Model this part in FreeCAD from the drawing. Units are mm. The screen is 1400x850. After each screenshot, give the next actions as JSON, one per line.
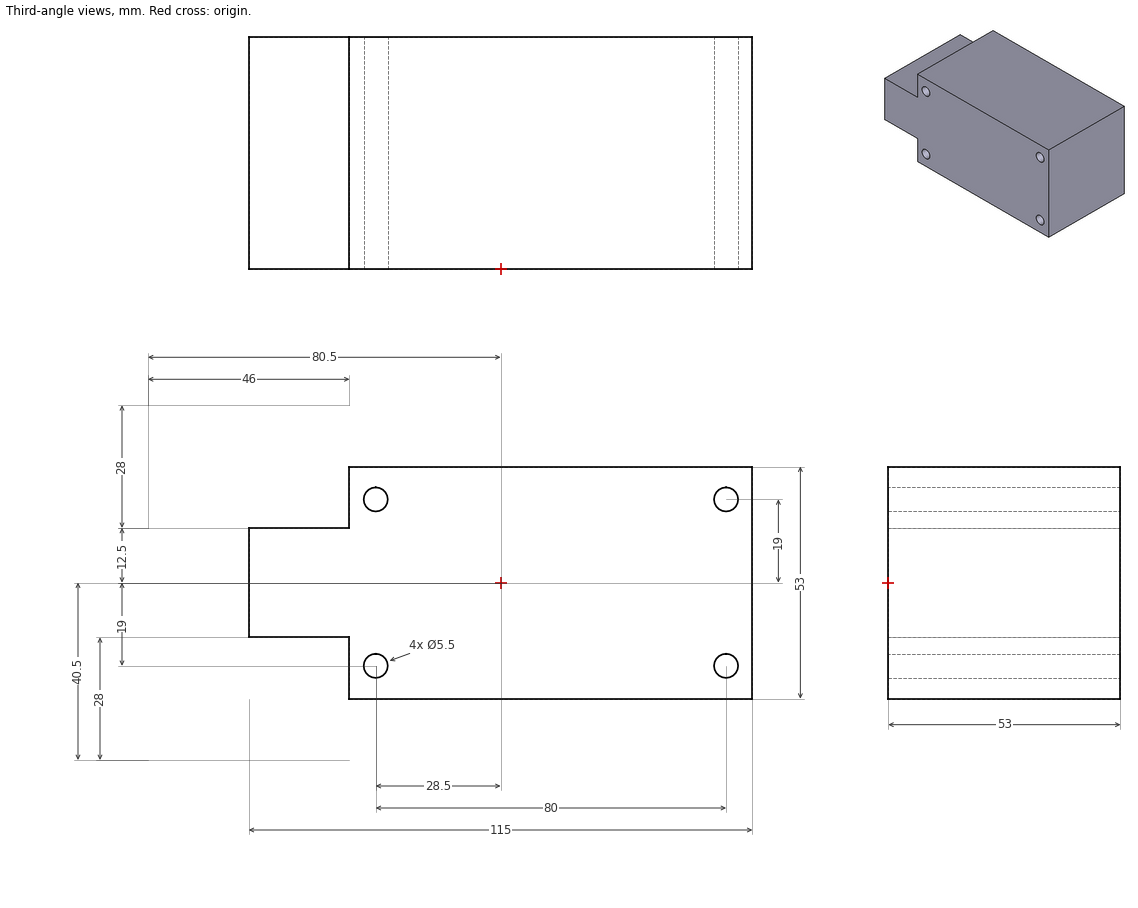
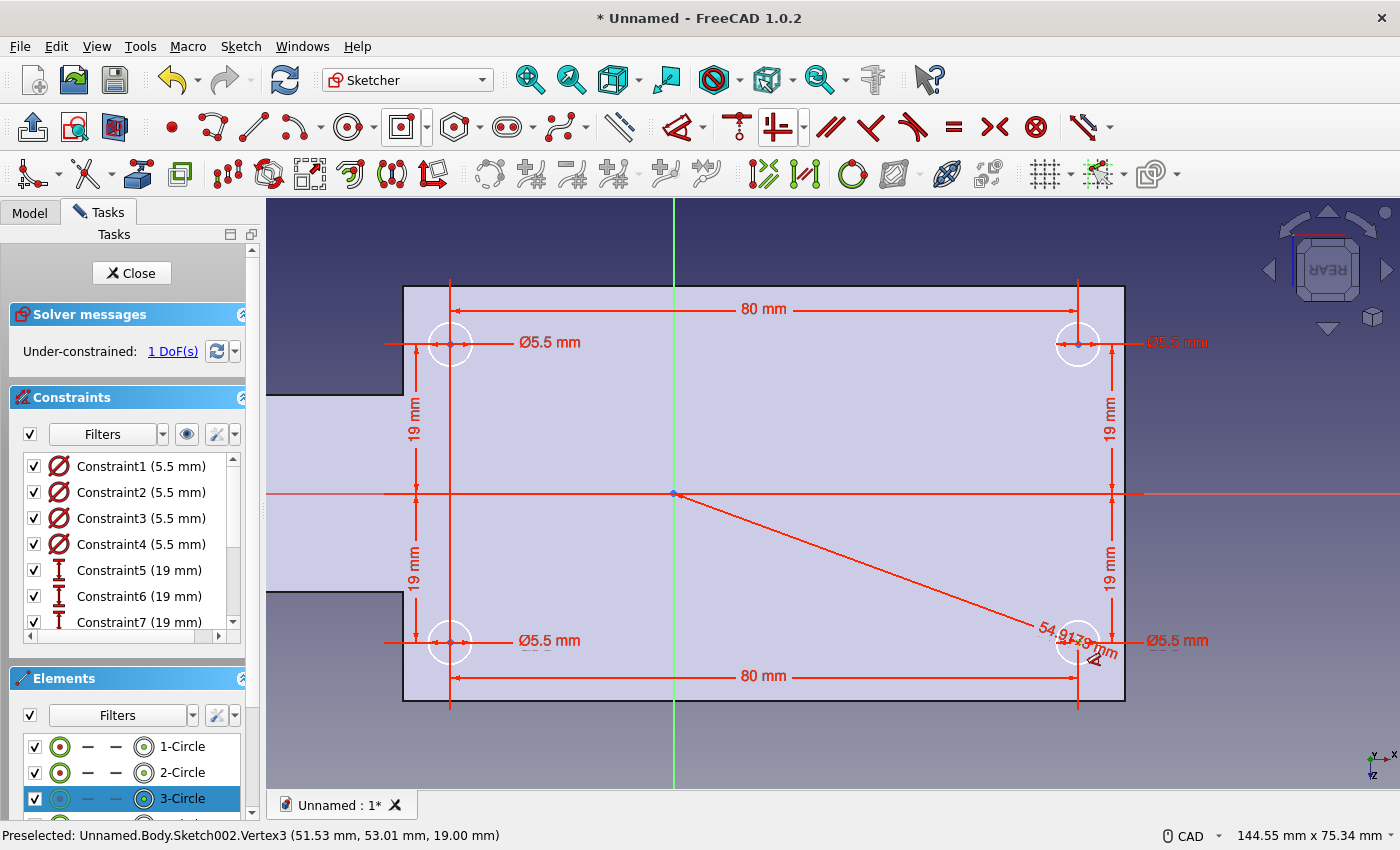
{"action": "left_click", "coordinate": [450, 643]}
{"action": "left_click", "coordinate": [620, 677]}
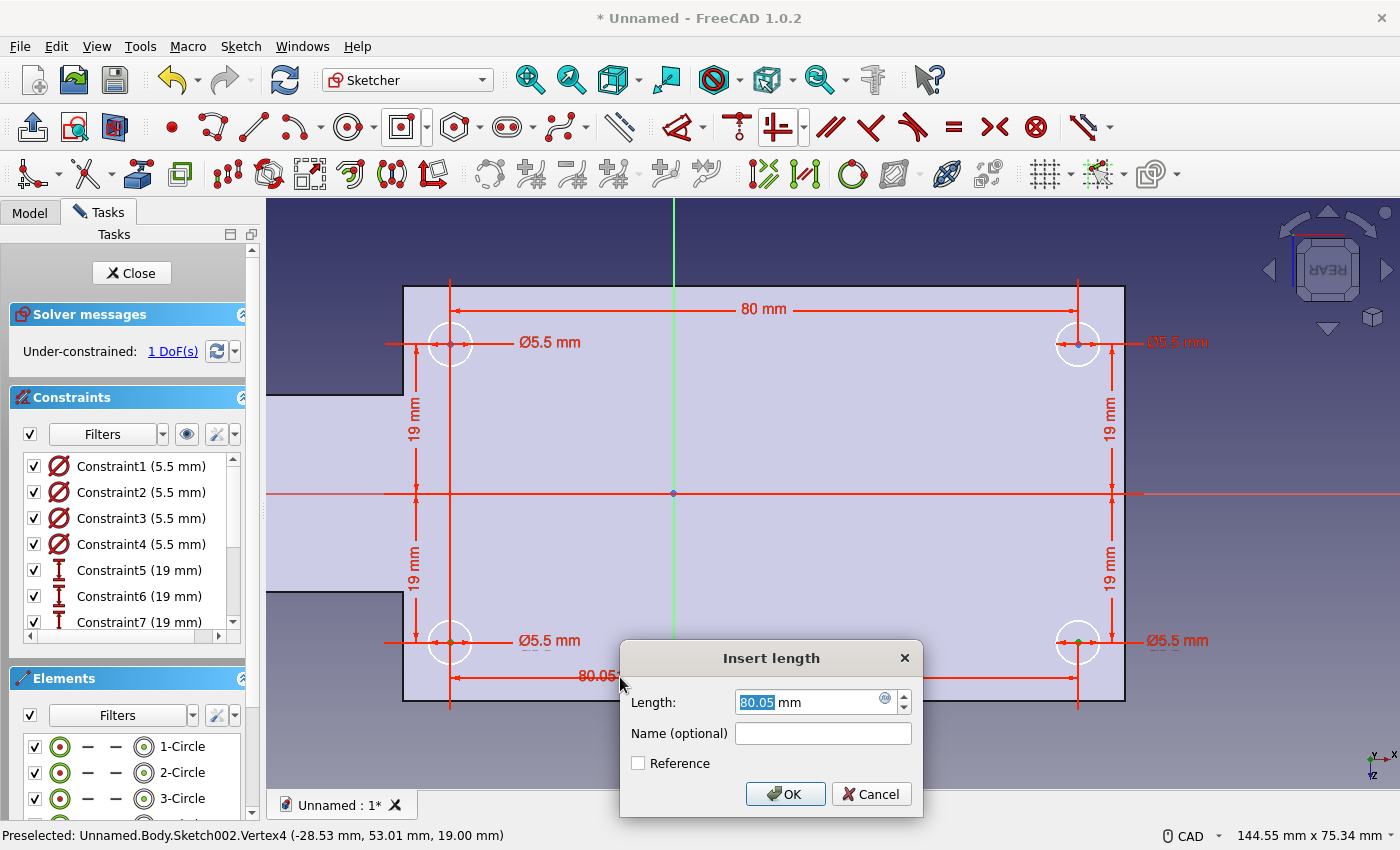
{"action": "type", "text": "80"}
{"action": "key", "text": "Return"}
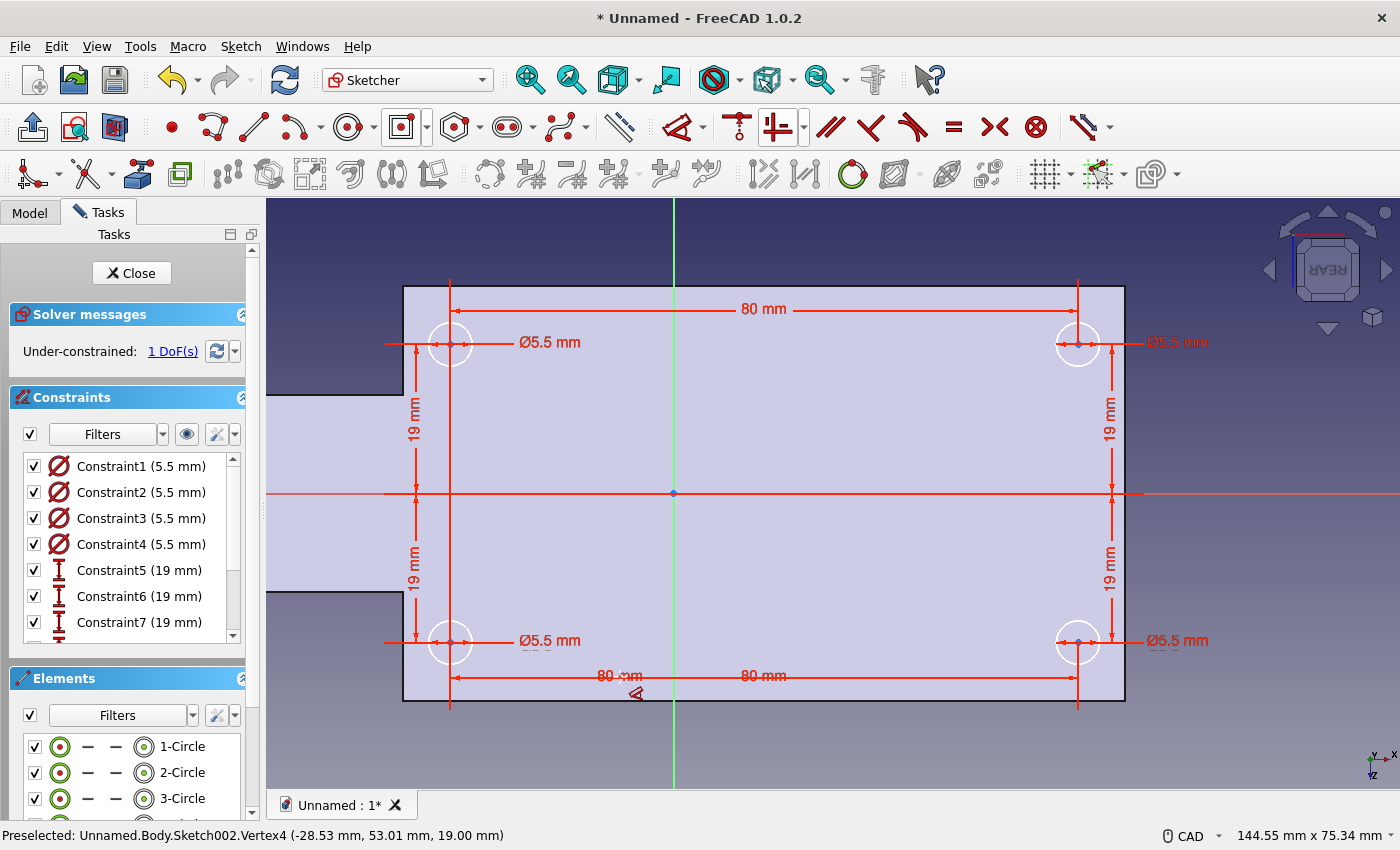
{"action": "left_click", "coordinate": [450, 344]}
{"action": "left_click", "coordinate": [562, 310]}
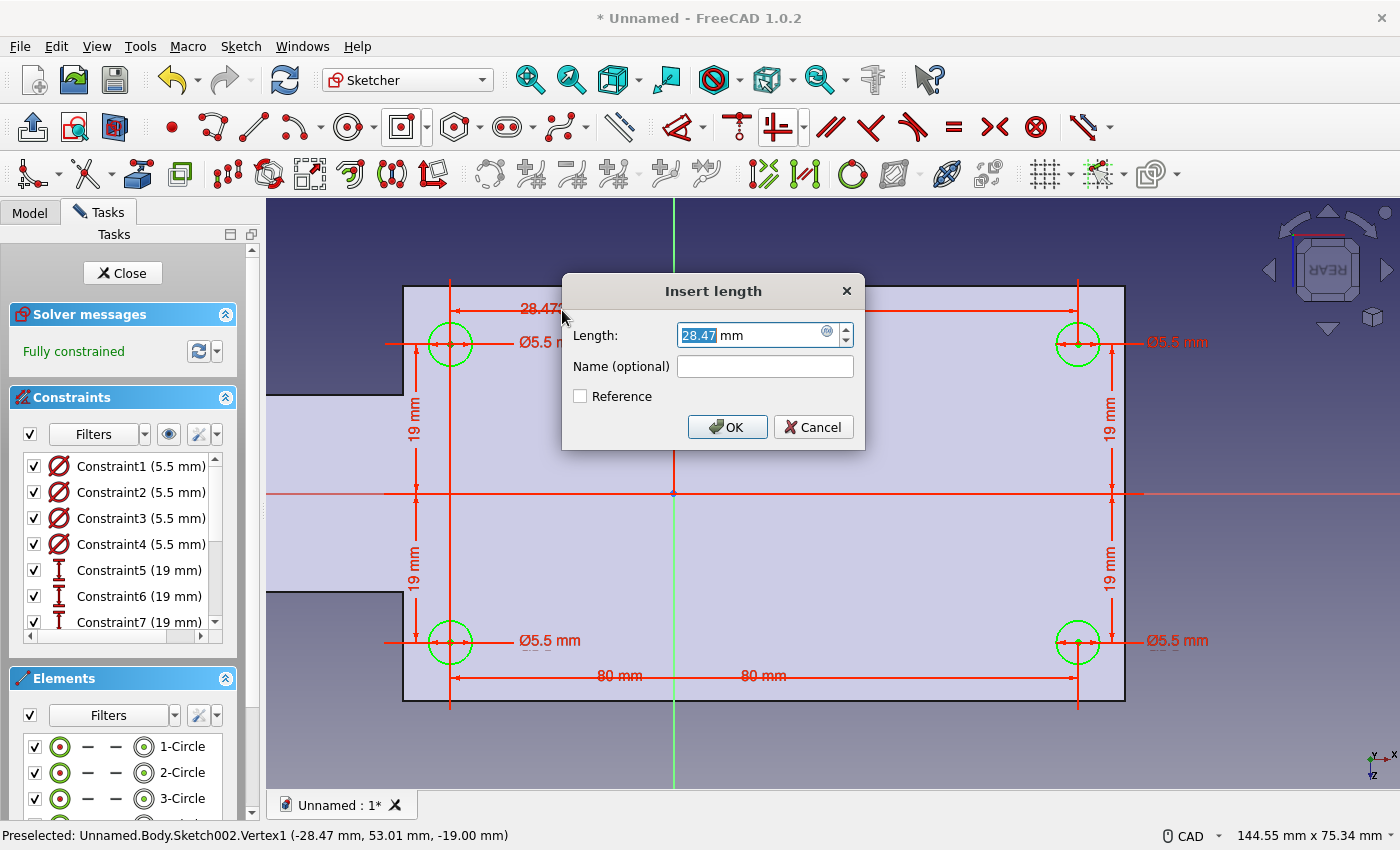
{"action": "type", "text": "28.5"}
{"action": "key", "text": "Return"}
{"action": "key", "text": "Escape"}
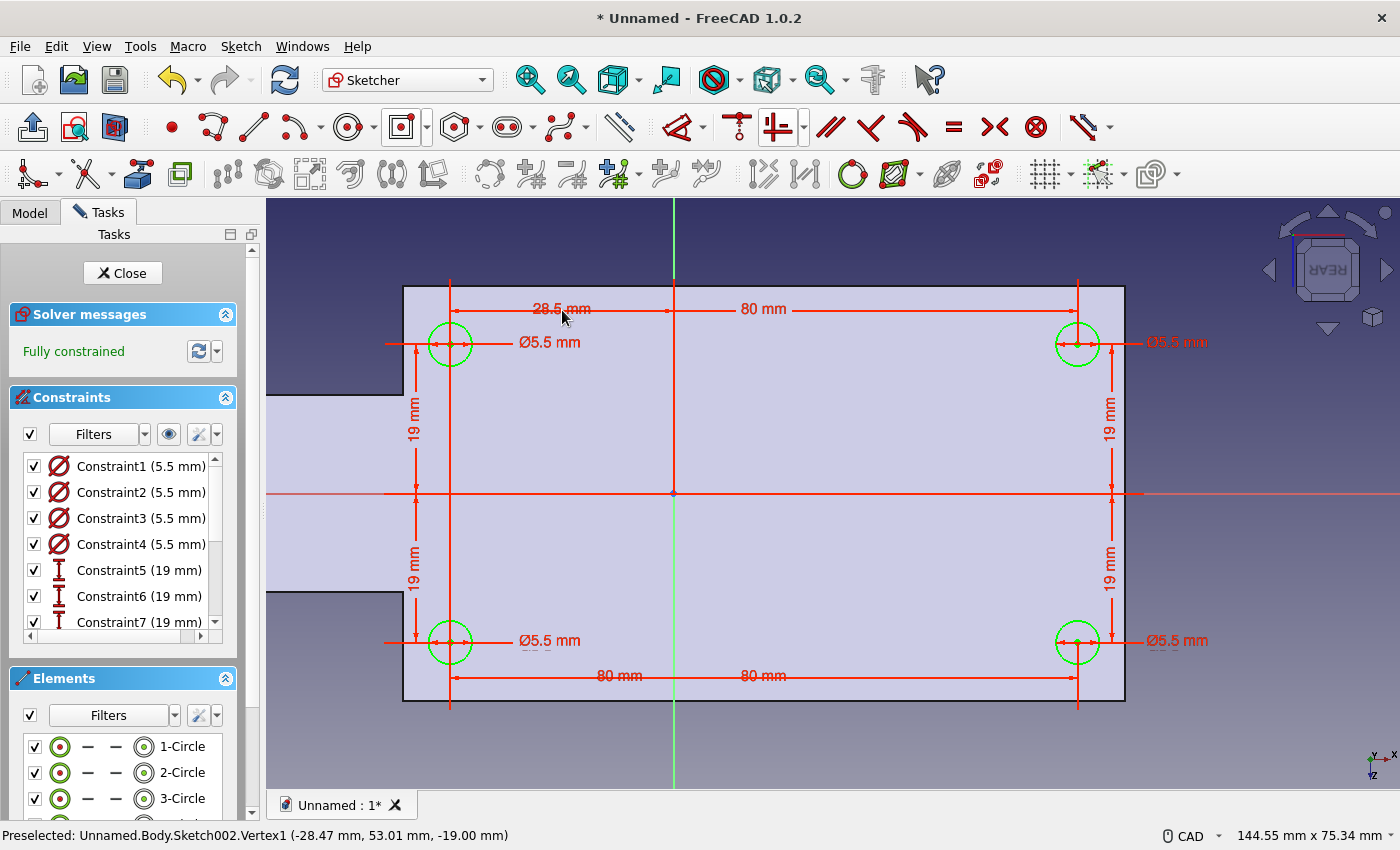
{"action": "left_click", "coordinate": [123, 273]}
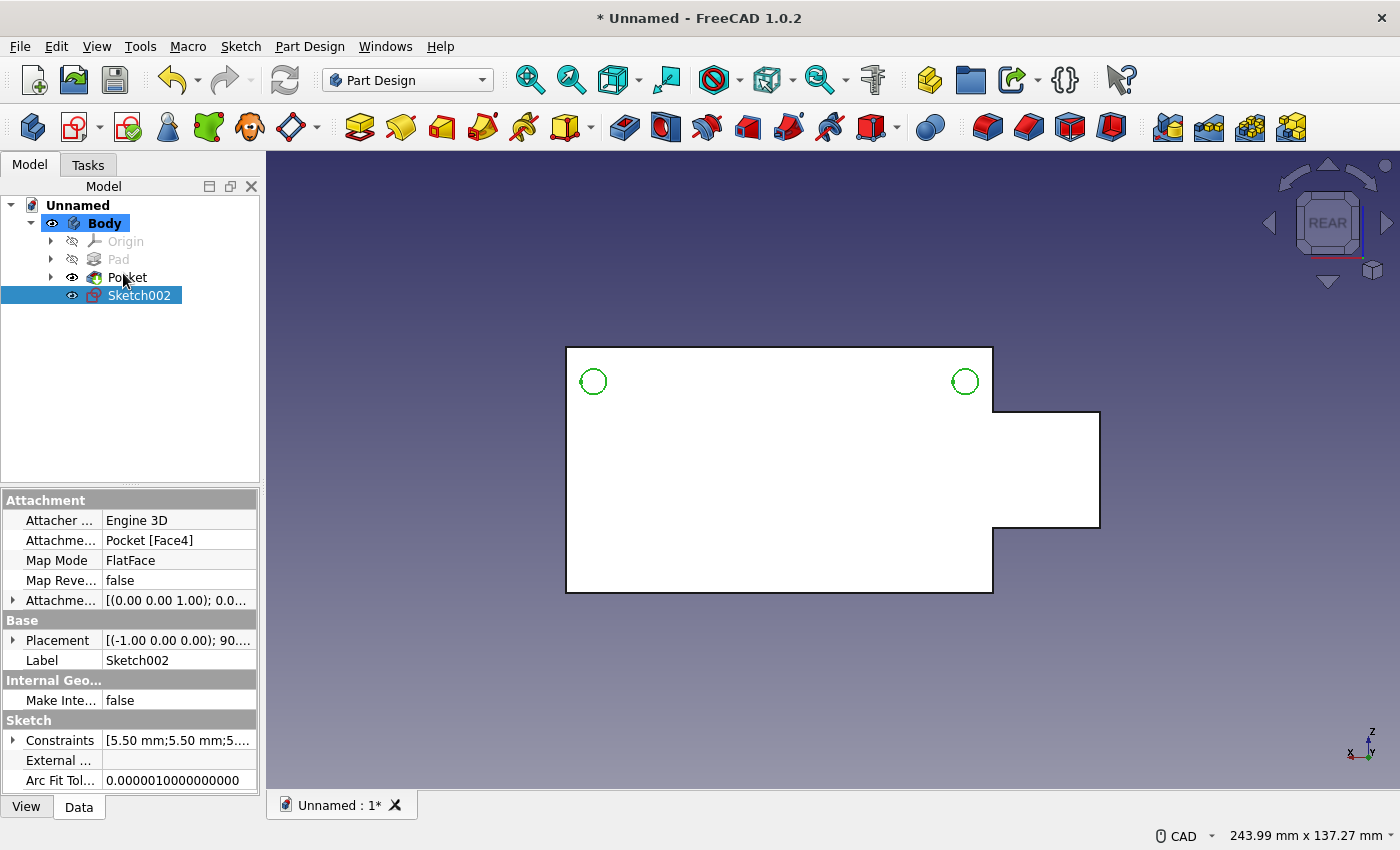
{"action": "left_click", "coordinate": [625, 128]}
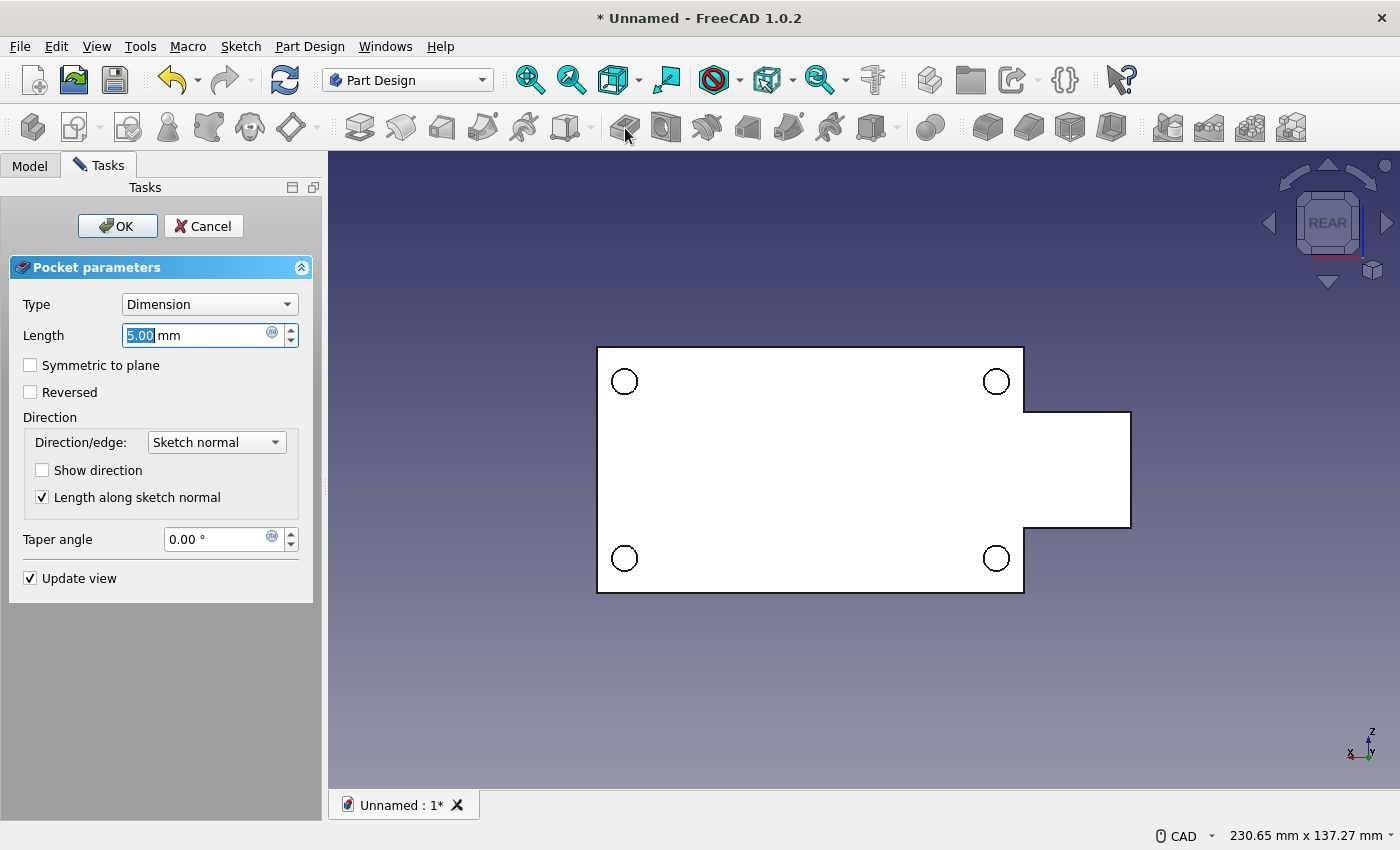
{"action": "left_click", "coordinate": [210, 304]}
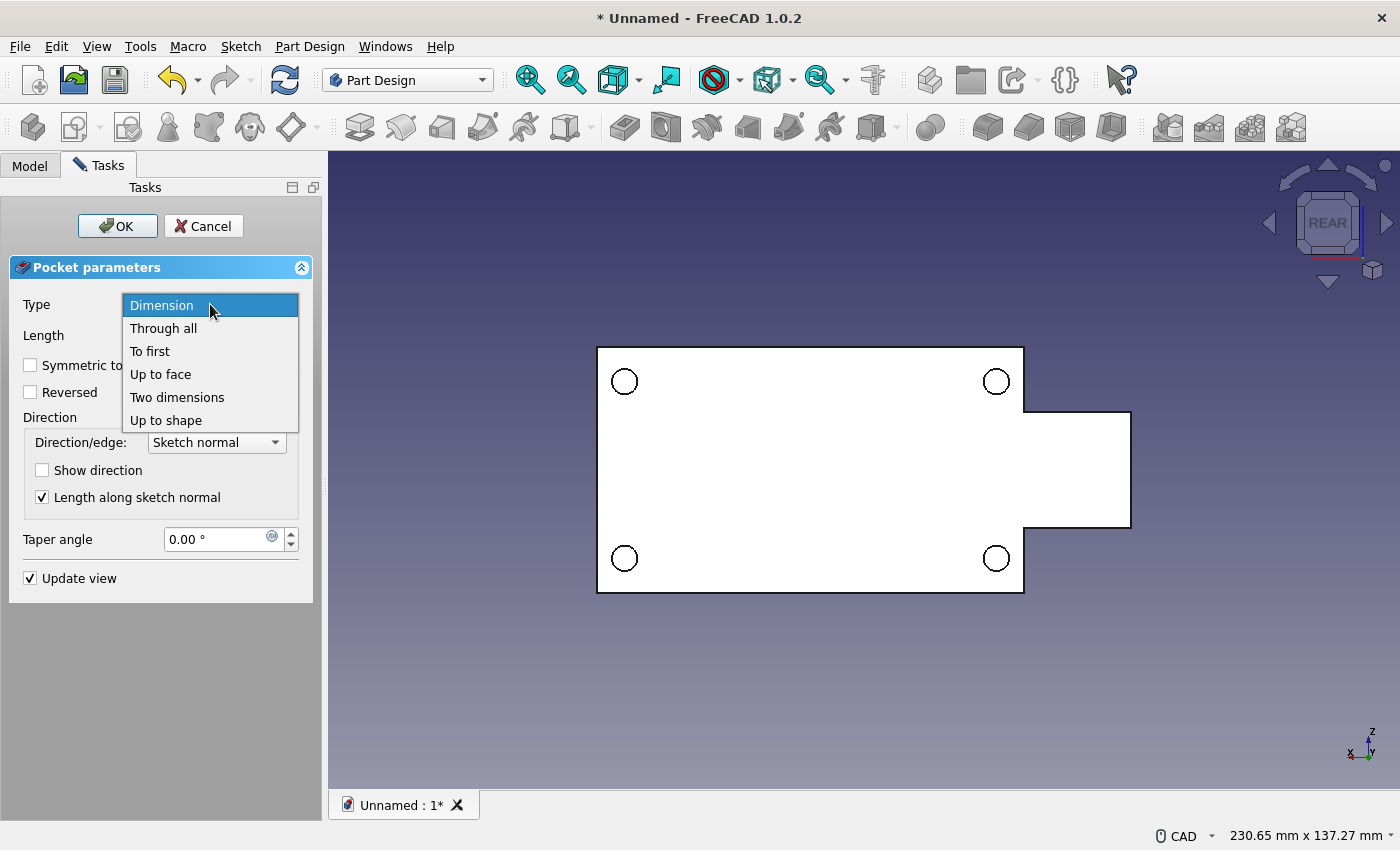
{"action": "left_click", "coordinate": [208, 328]}